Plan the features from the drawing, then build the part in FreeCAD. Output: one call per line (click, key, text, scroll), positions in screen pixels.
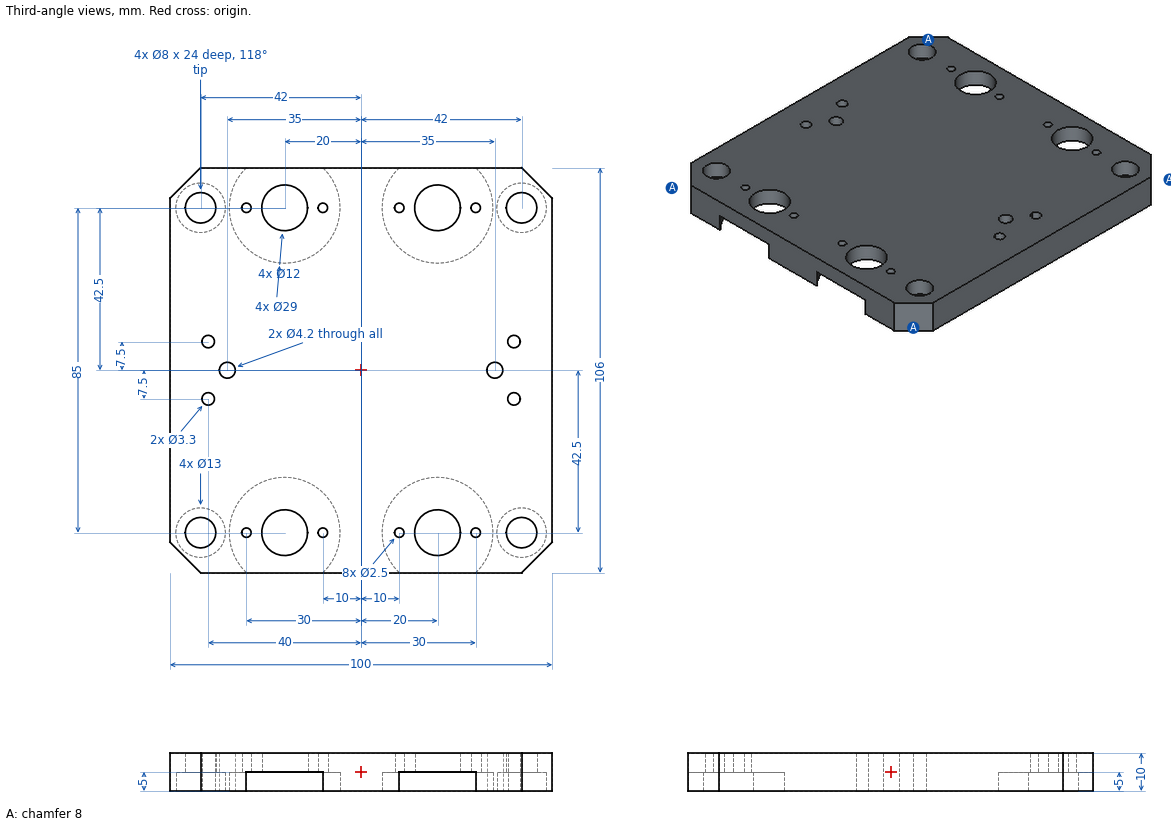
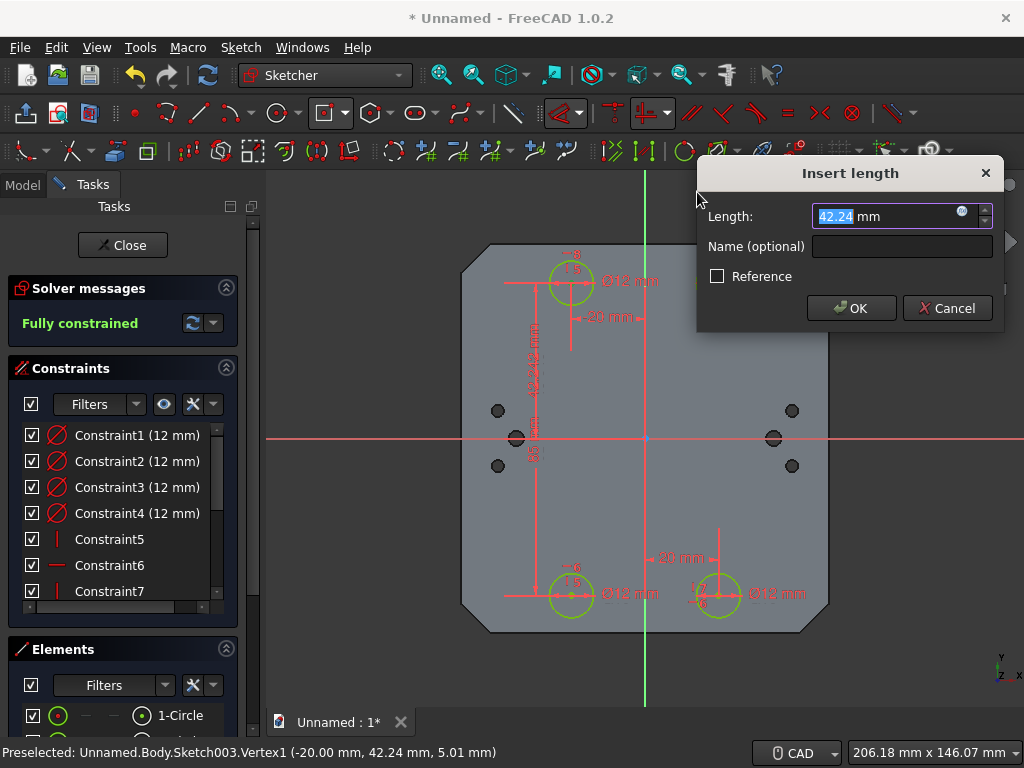
text(42.5)
key(Return)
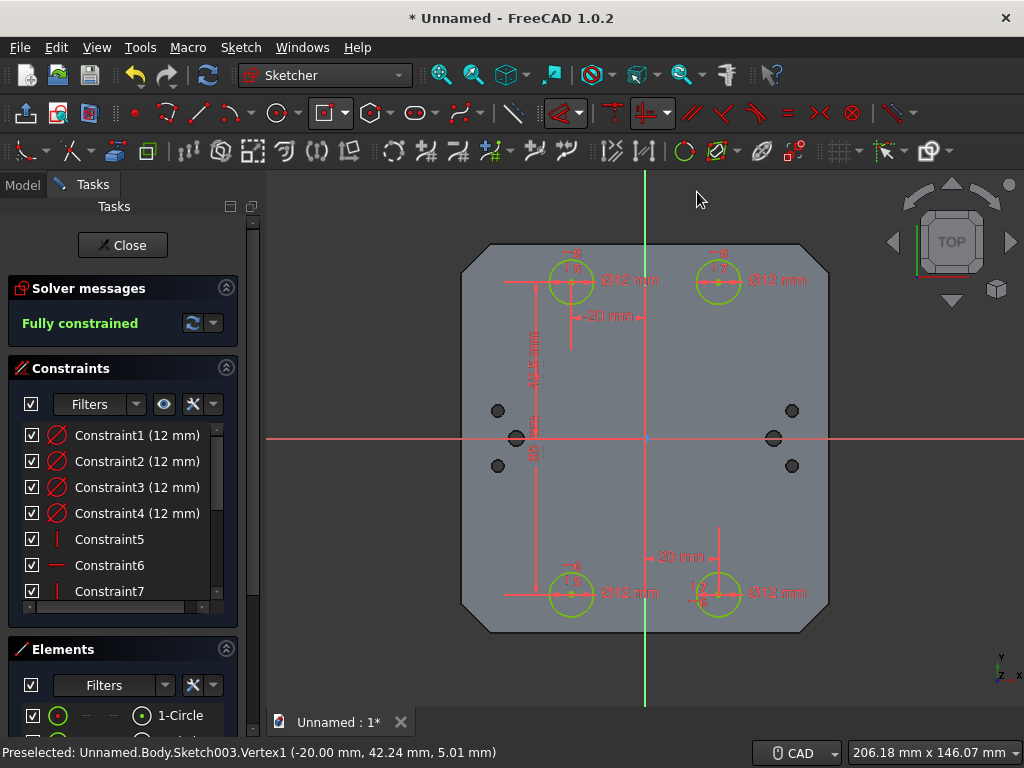
click(123, 245)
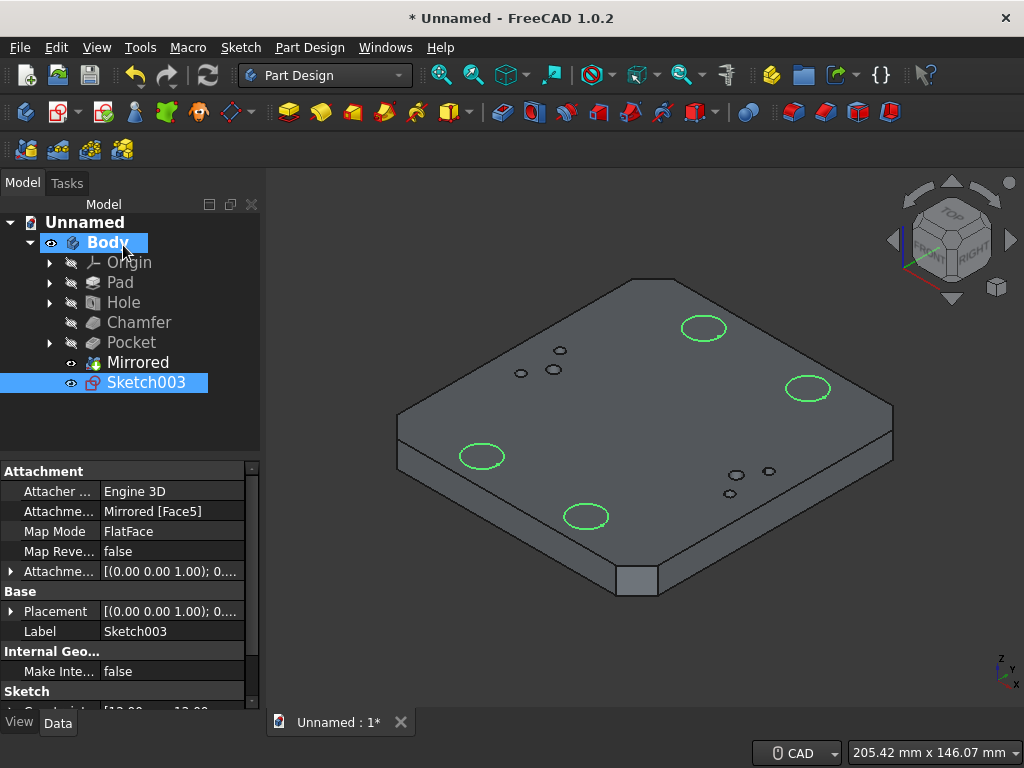
click(504, 112)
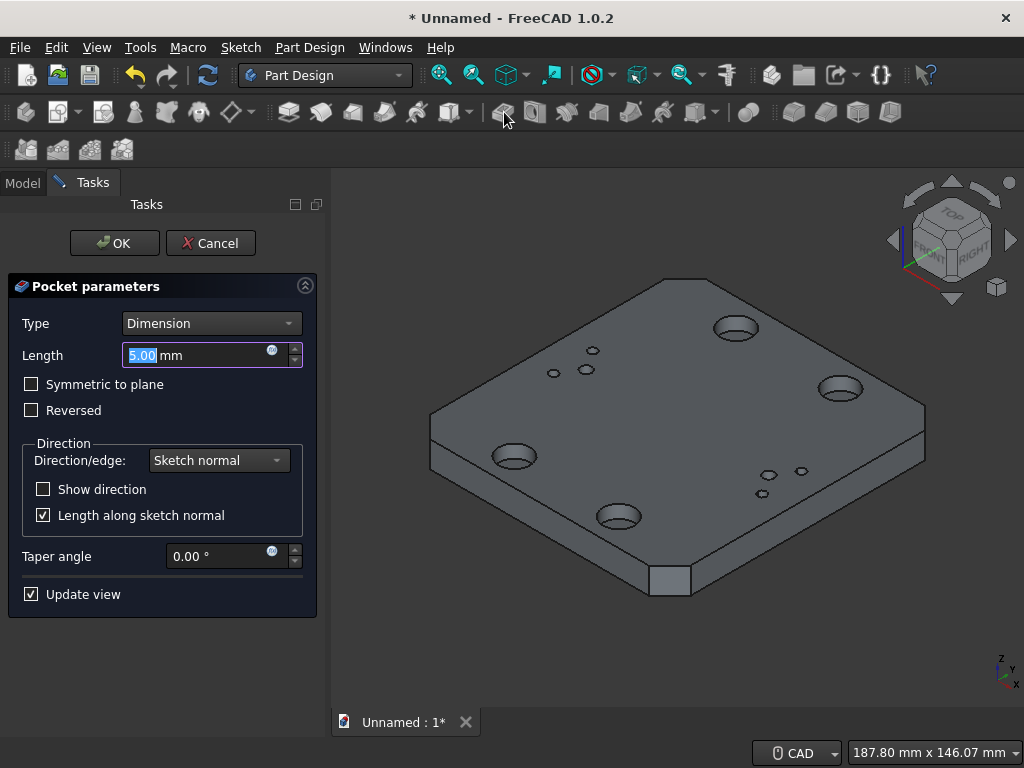
click(212, 324)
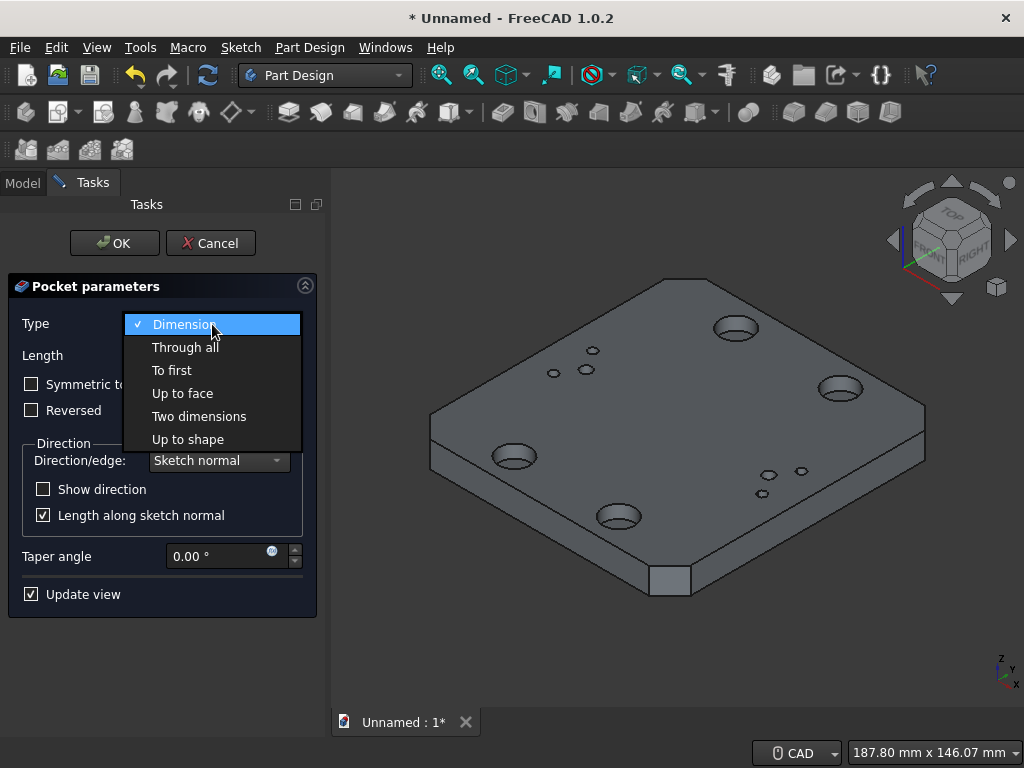
click(212, 348)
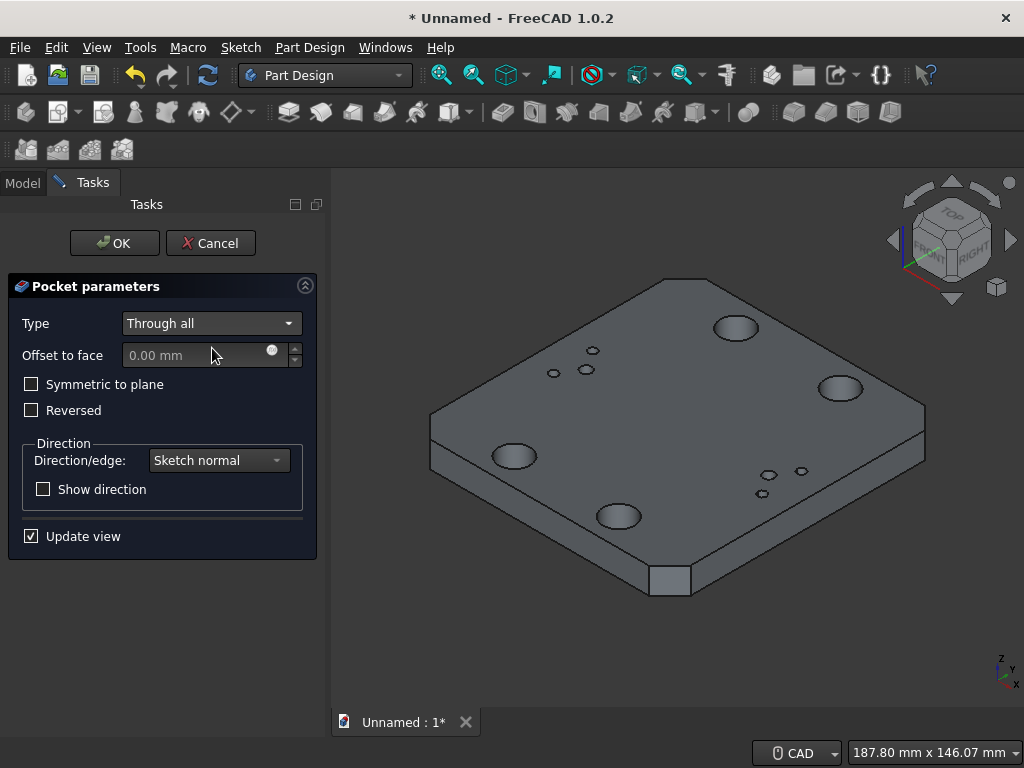
click(115, 243)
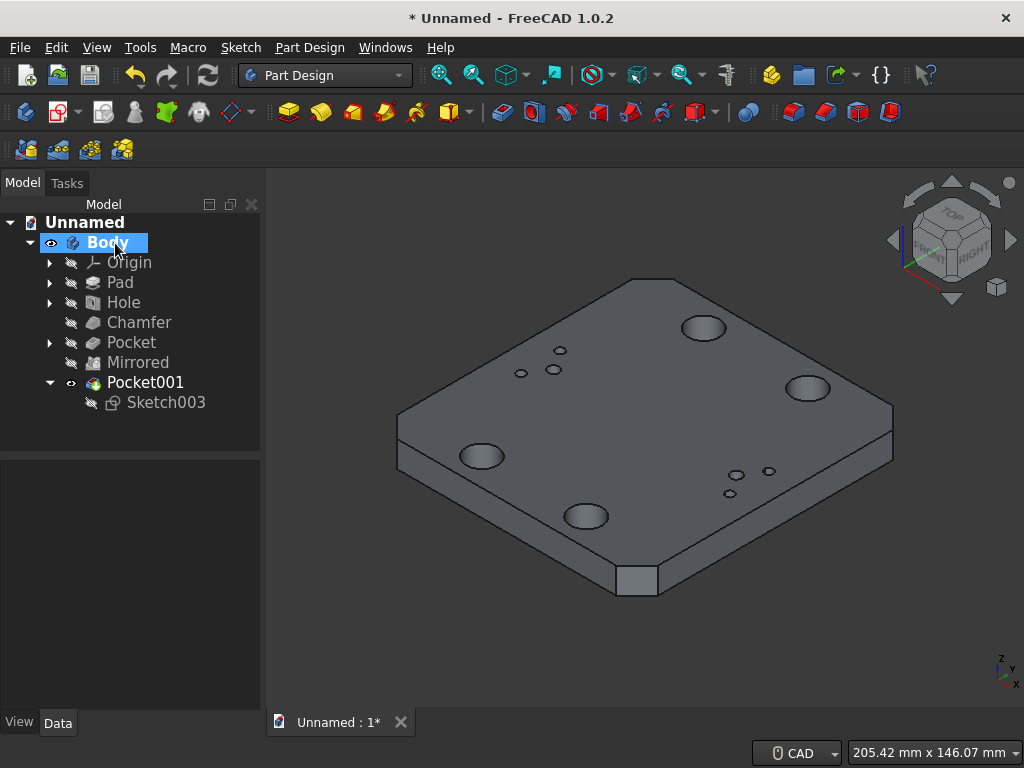
click(645, 421)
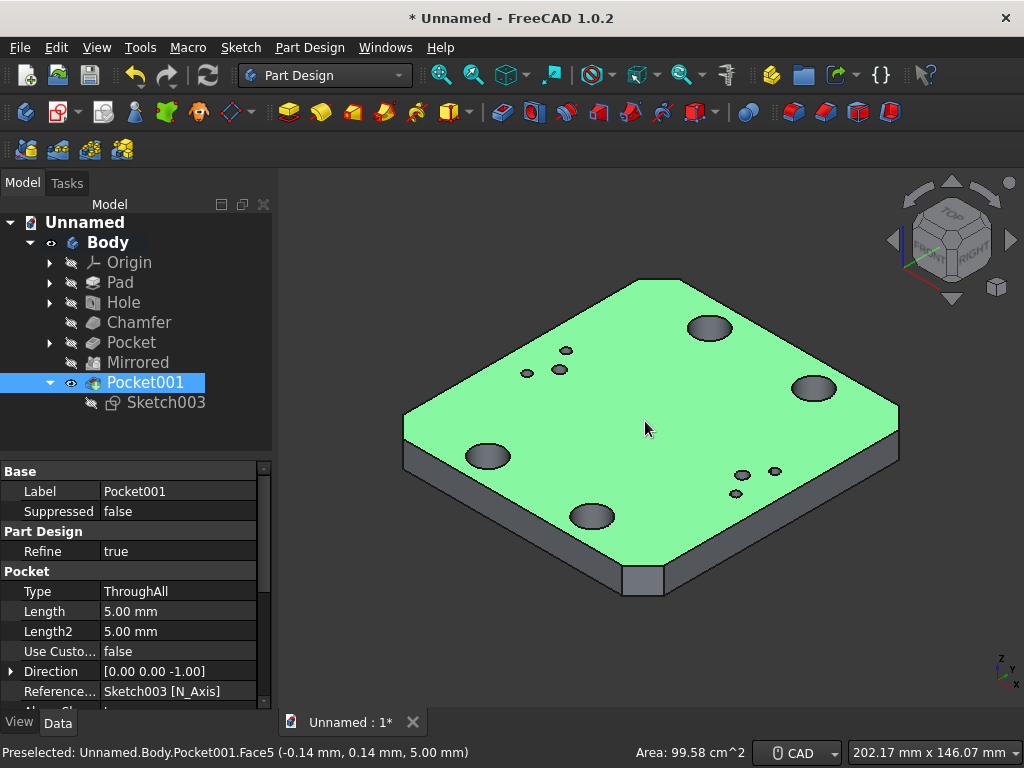
click(58, 112)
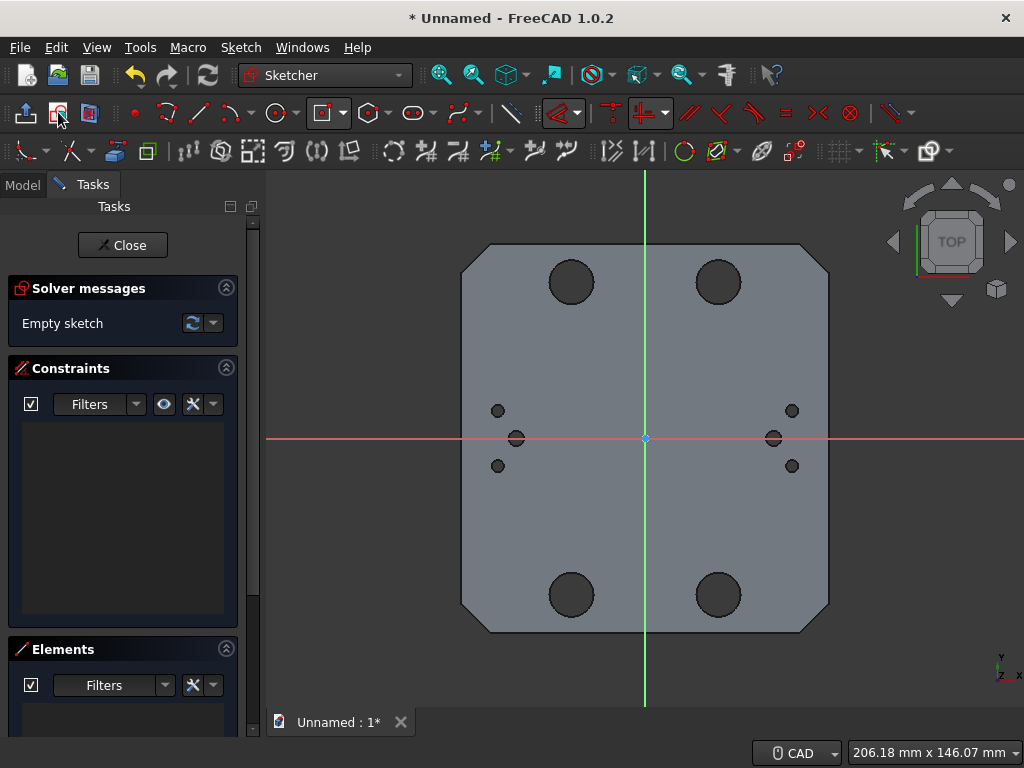
click(276, 114)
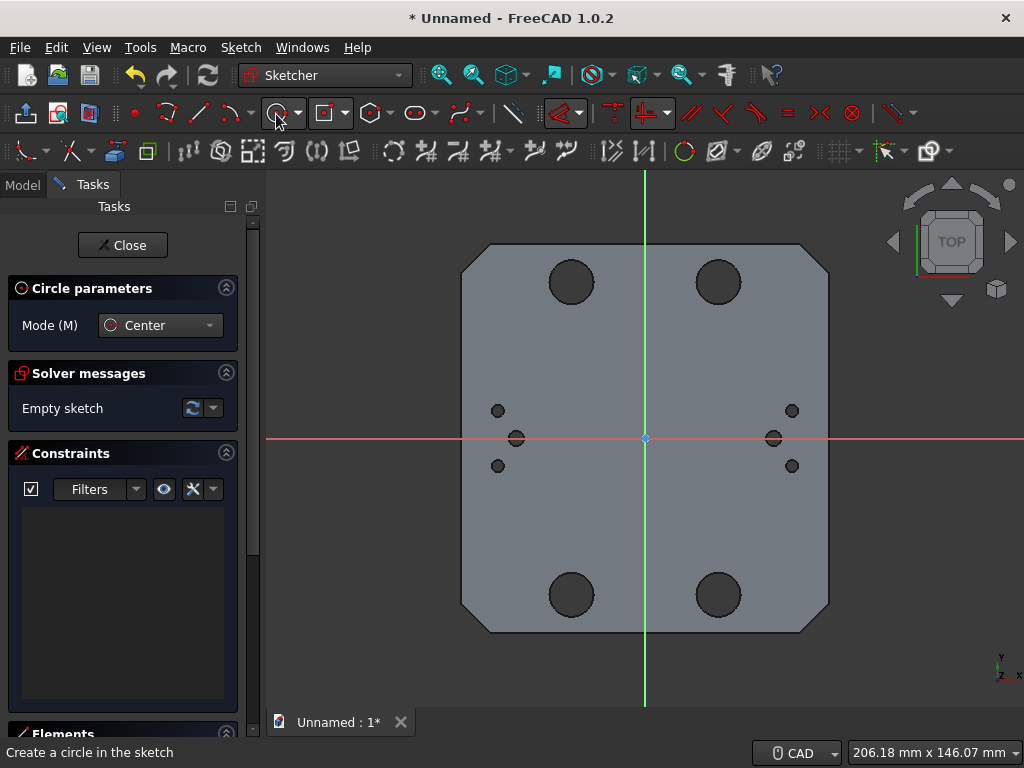
scroll(682, 595, up, 8)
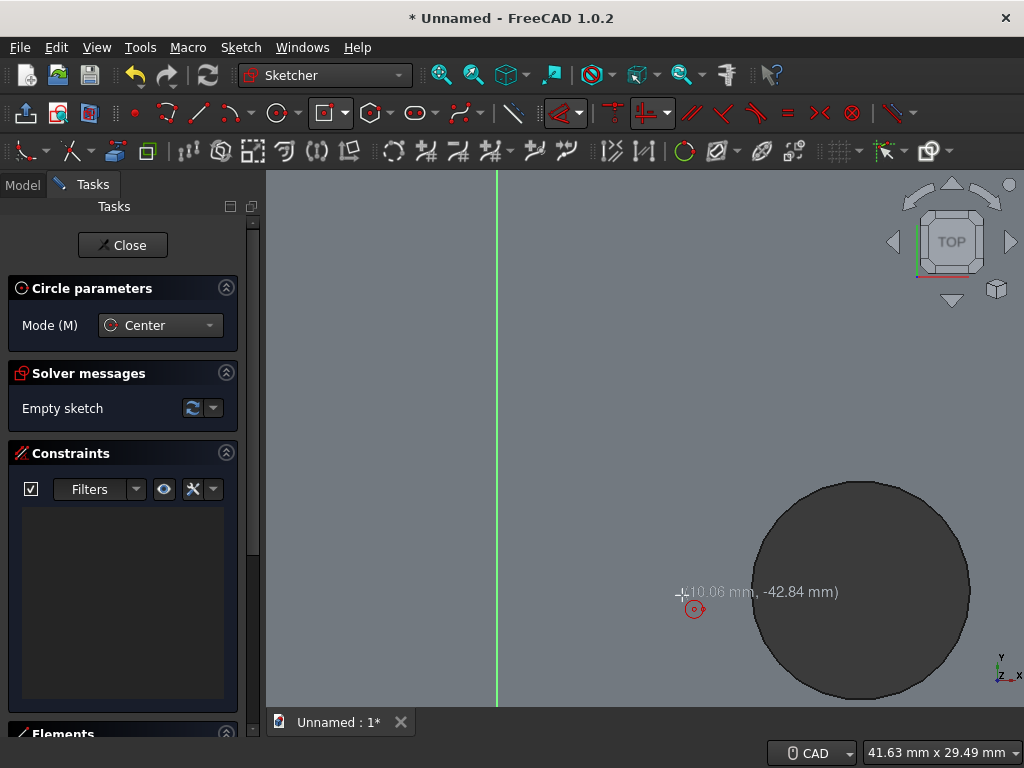
scroll(597, 596, down, 8)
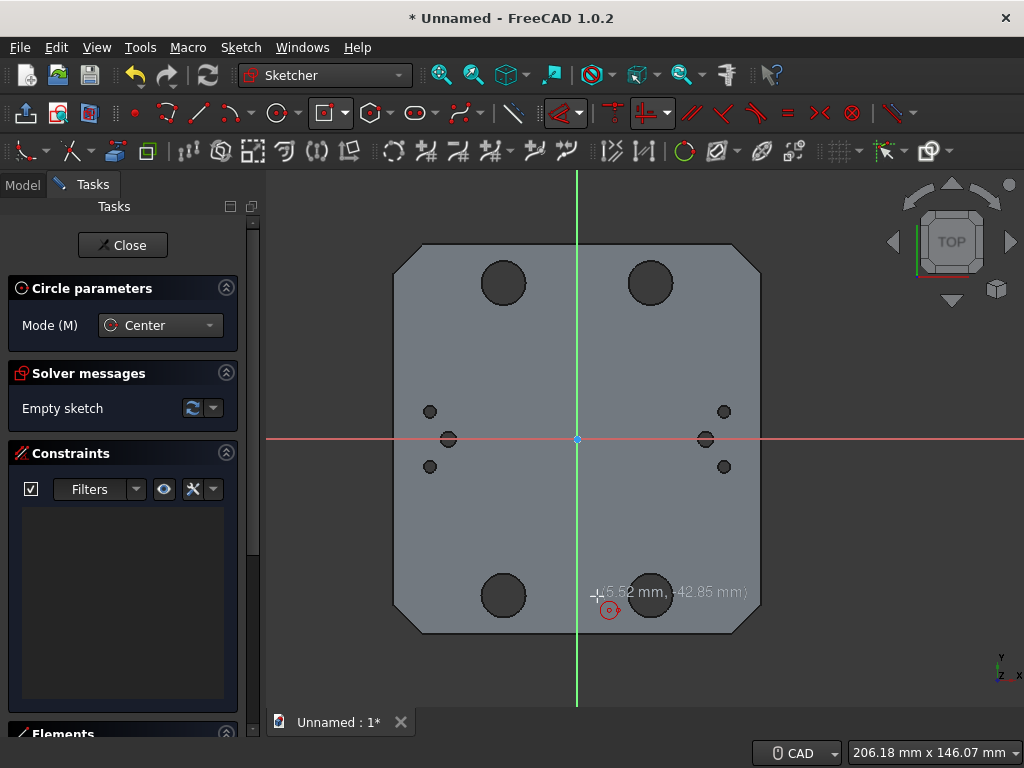
click(614, 596)
move(617, 592)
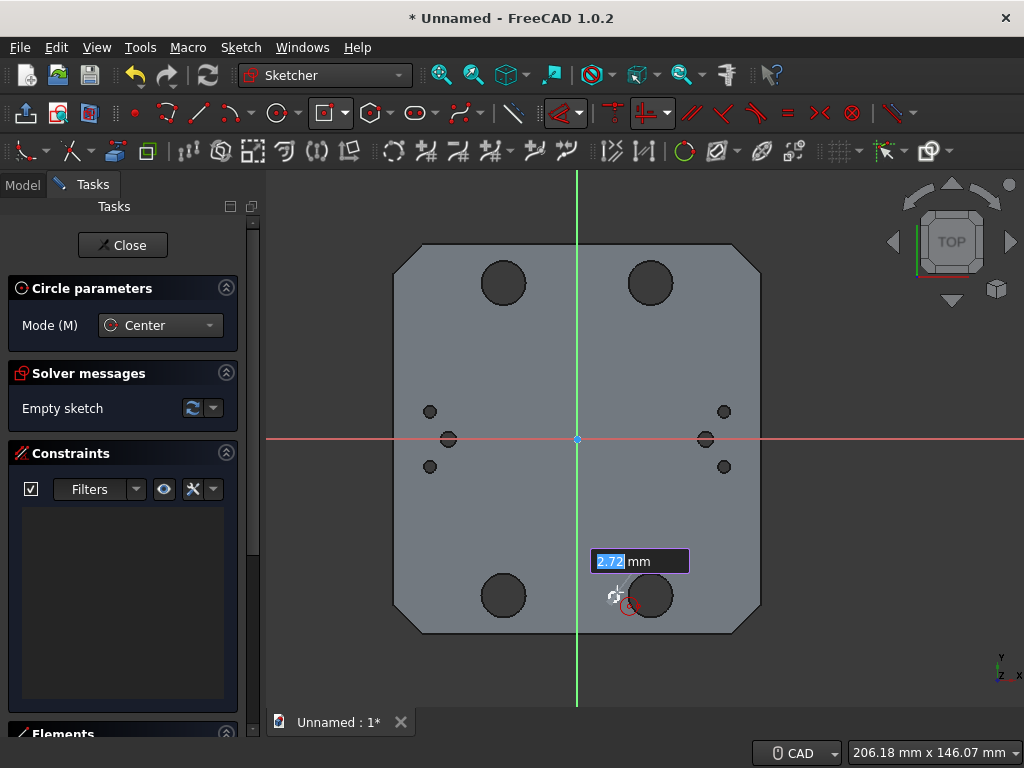
text(2.5)
key(Return)